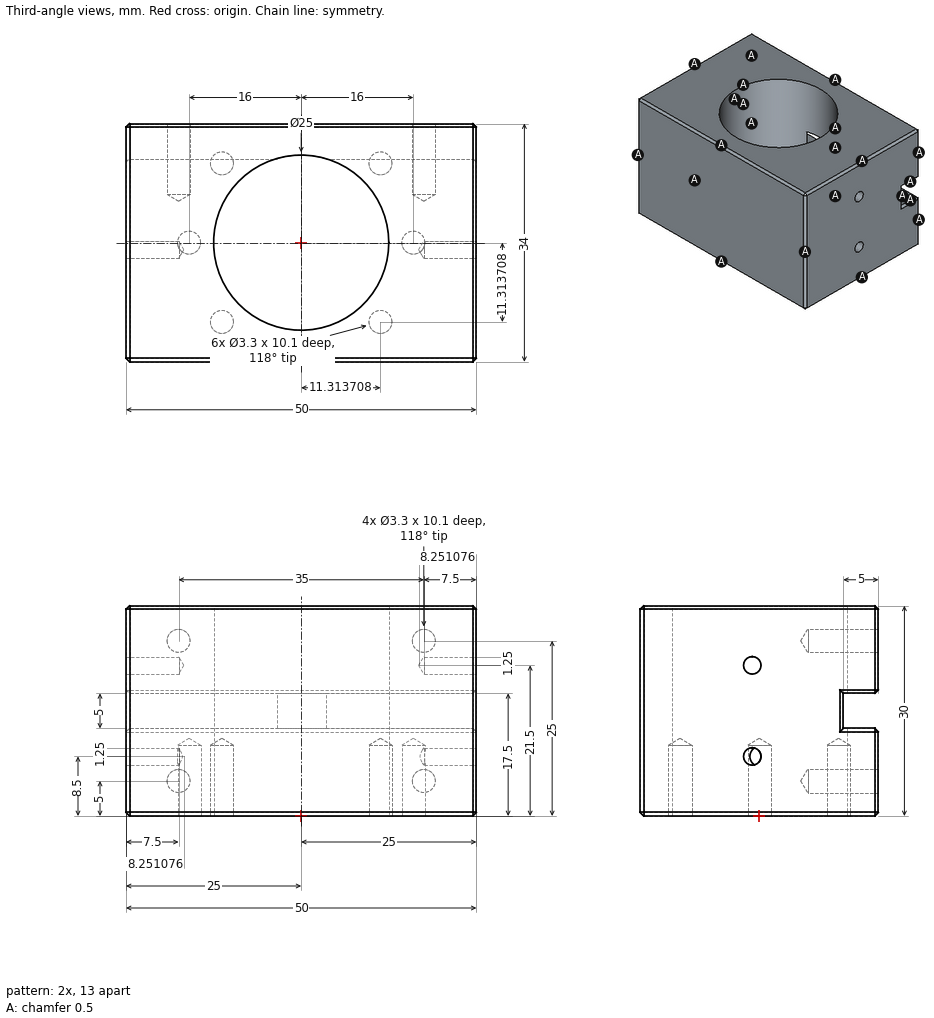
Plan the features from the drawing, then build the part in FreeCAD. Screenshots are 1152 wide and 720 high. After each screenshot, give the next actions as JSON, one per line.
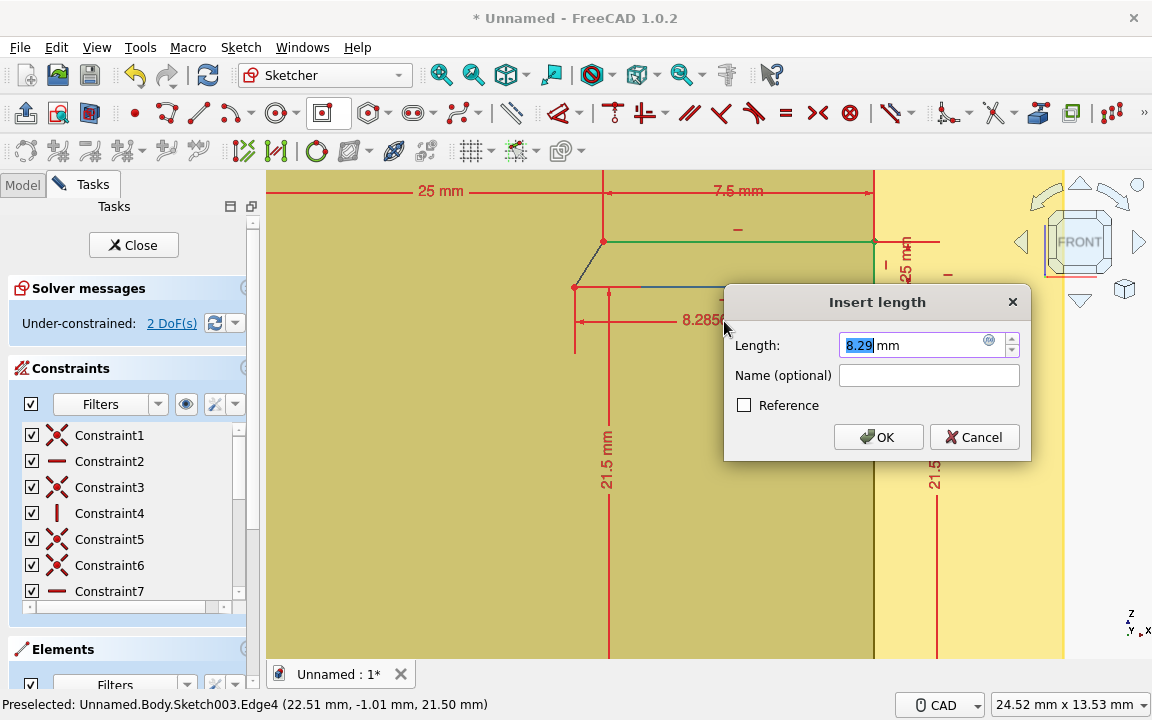
{"action": "type", "text": "8.251076"}
{"action": "key", "text": "Return"}
{"action": "key", "text": "Escape"}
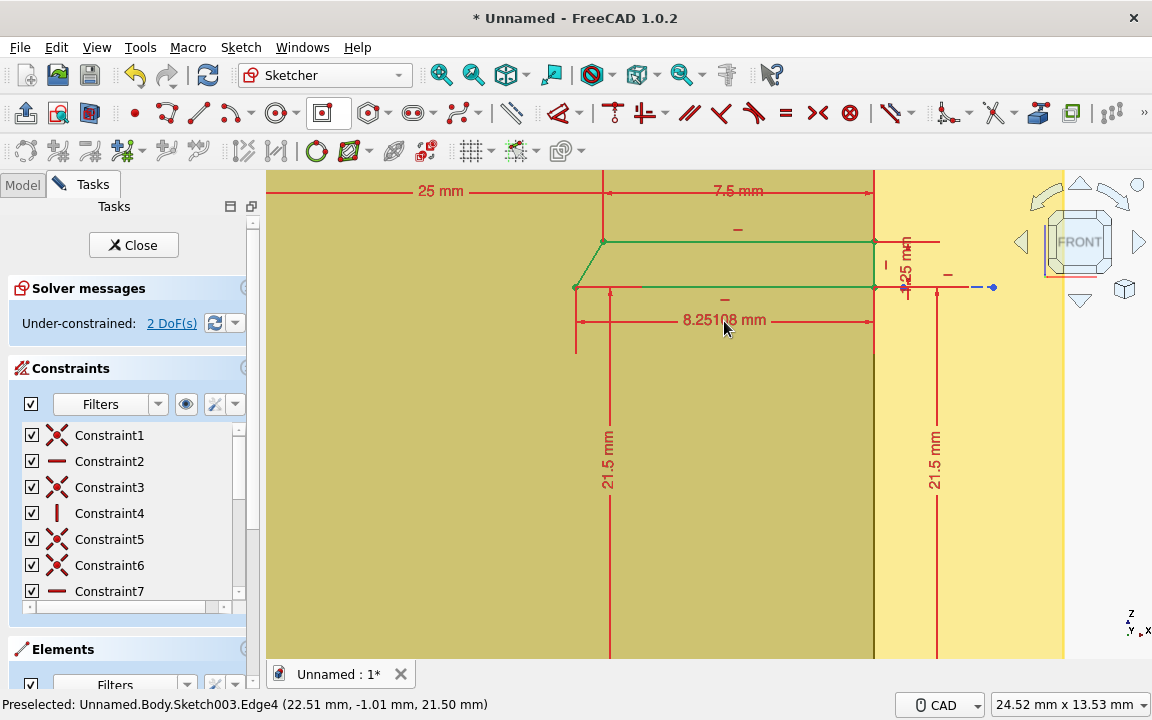
{"action": "left_click", "coordinate": [134, 245]}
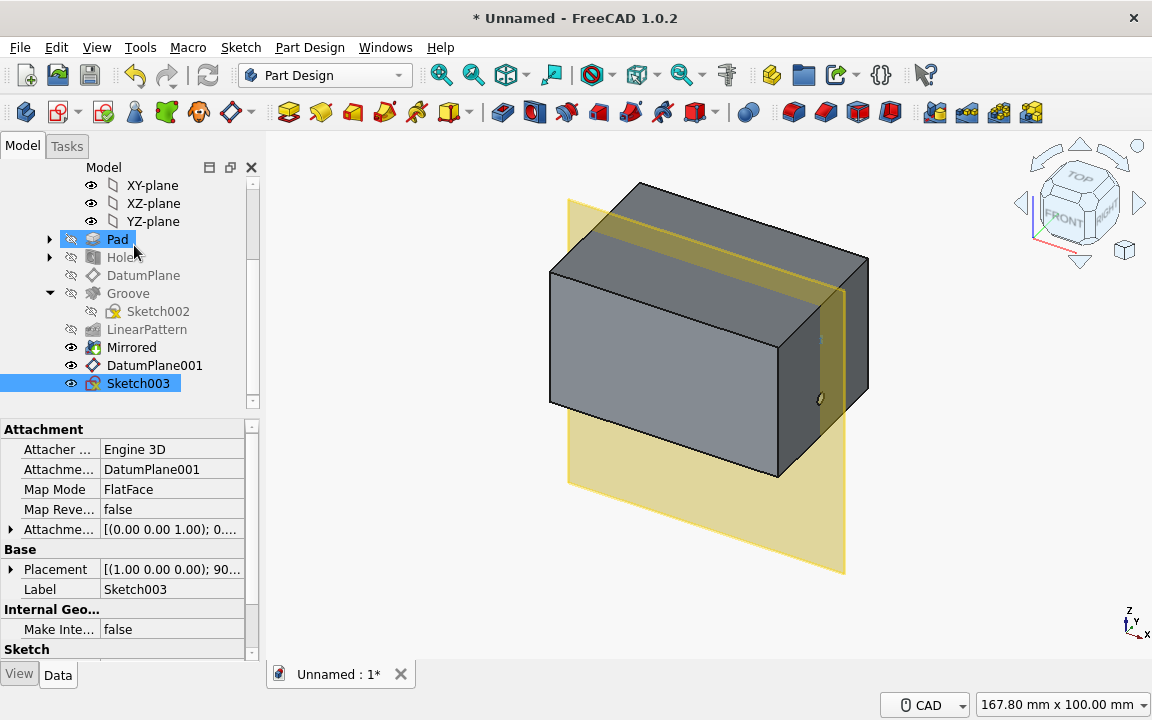
{"action": "left_click", "coordinate": [568, 112]}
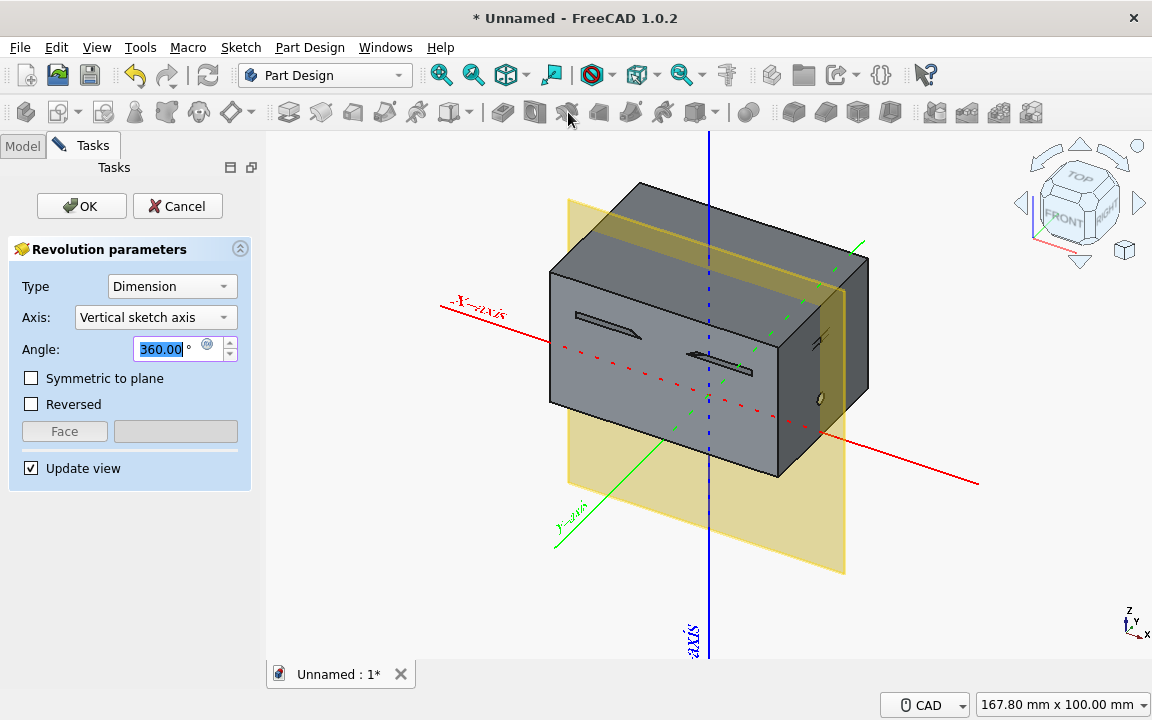
{"action": "left_click", "coordinate": [156, 318]}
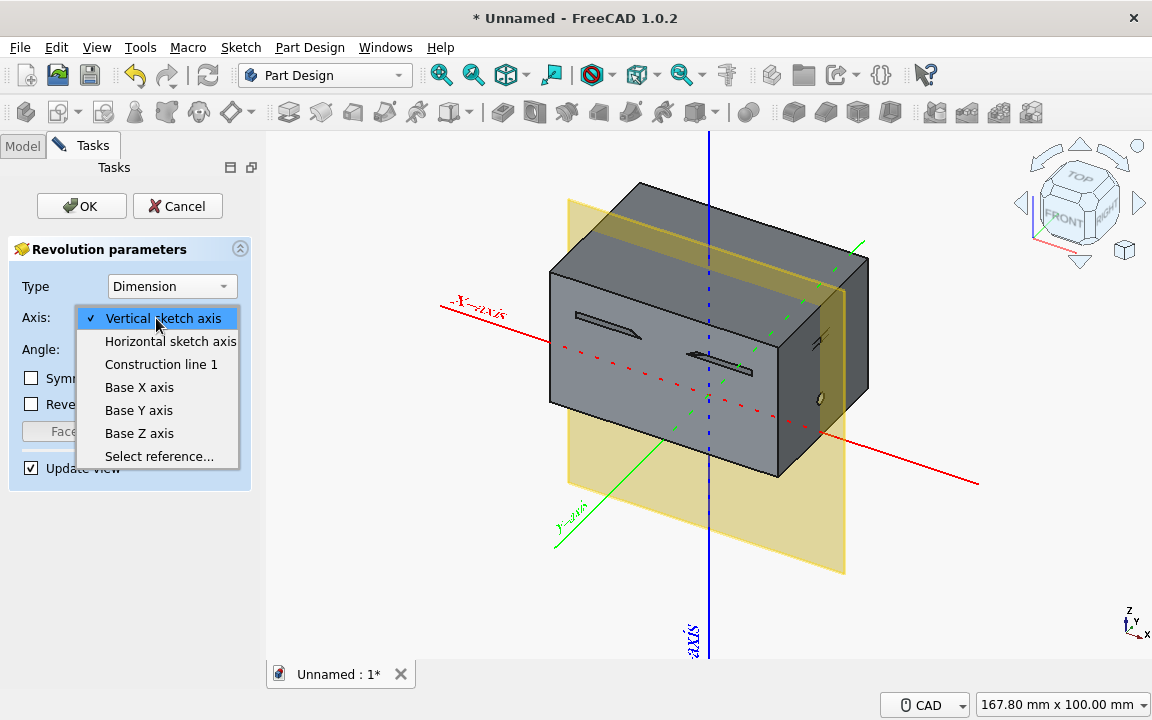
{"action": "left_click", "coordinate": [156, 364]}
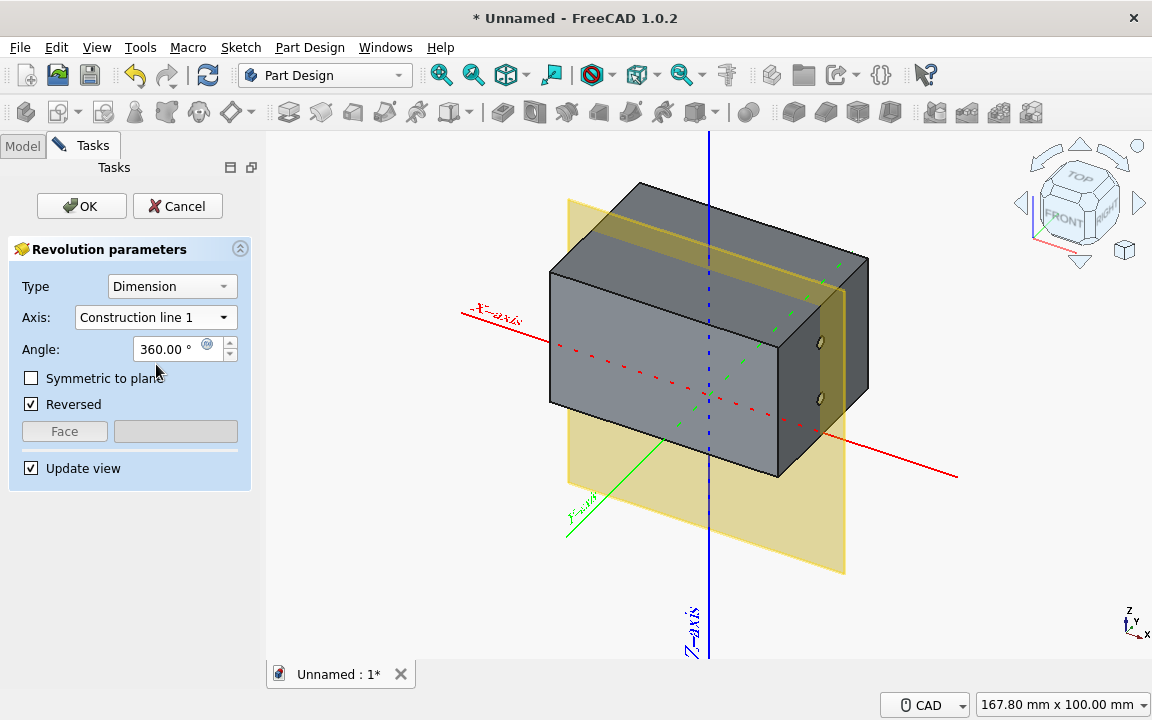
{"action": "left_click", "coordinate": [82, 206]}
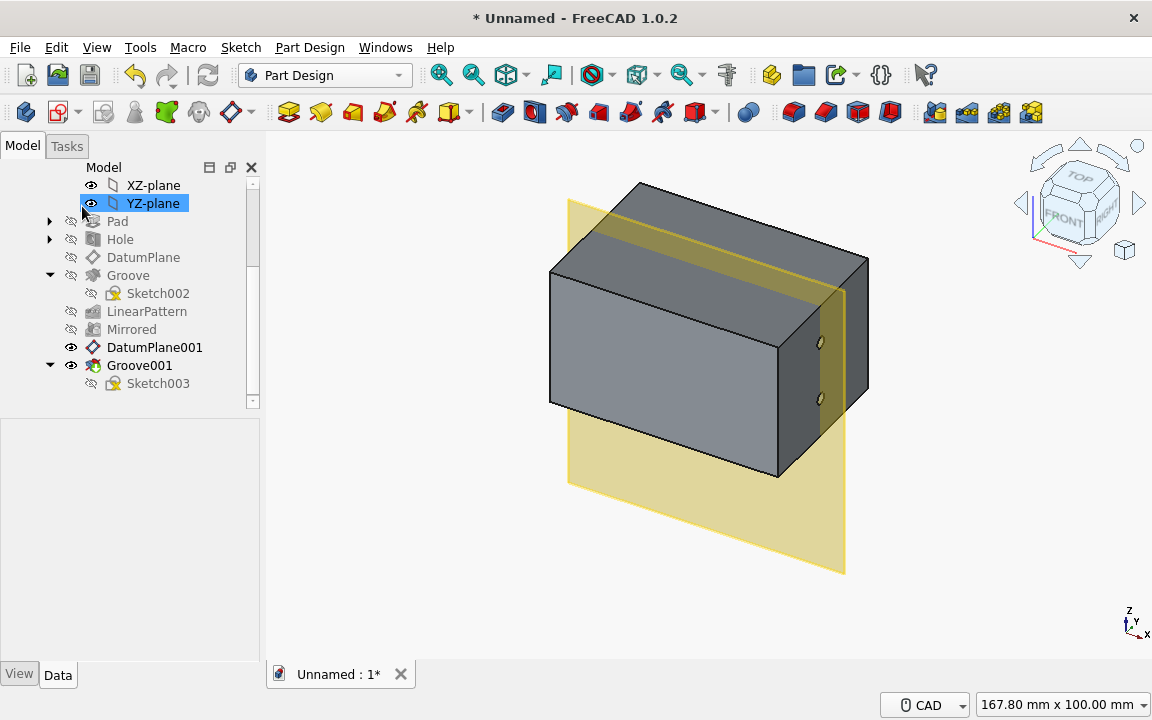
{"action": "left_click", "coordinate": [116, 347]}
{"action": "key", "text": "space"}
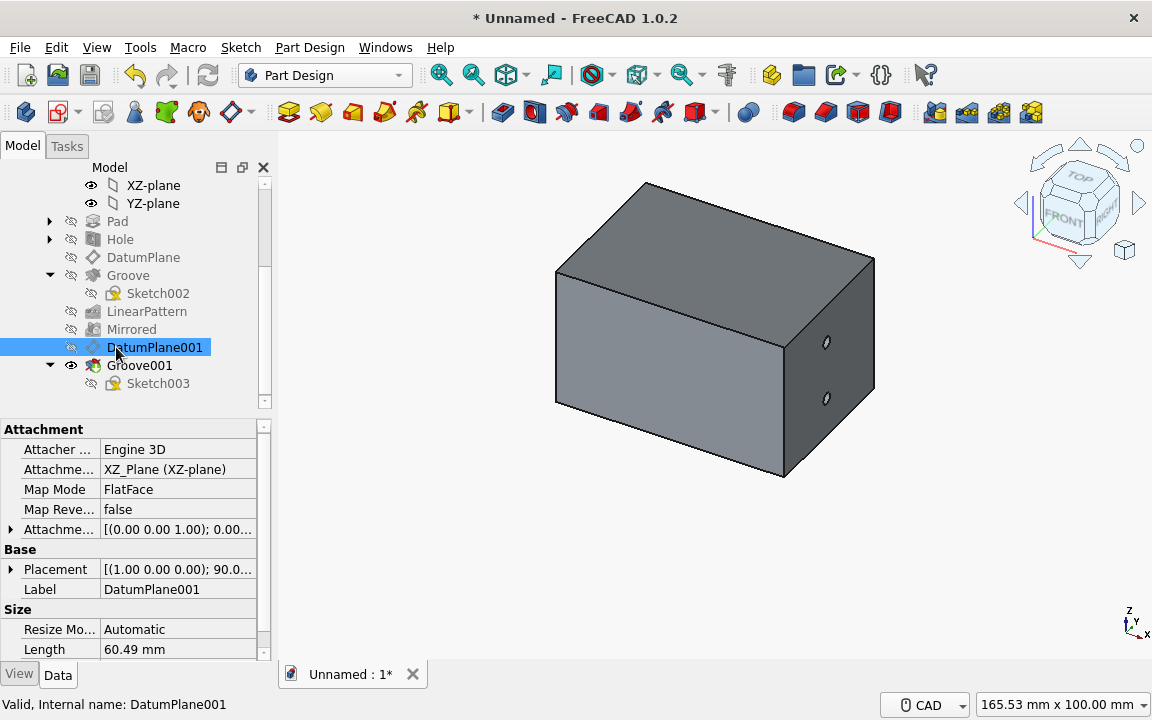
{"action": "left_click", "coordinate": [748, 275]}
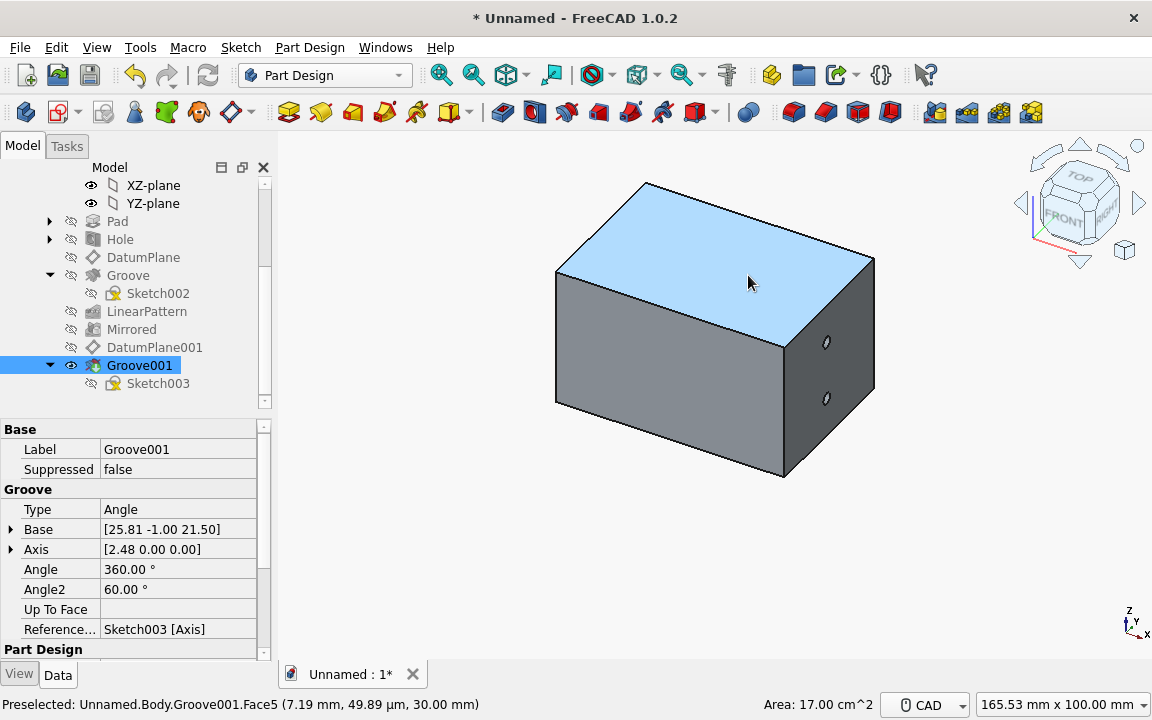
{"action": "left_click", "coordinate": [58, 112]}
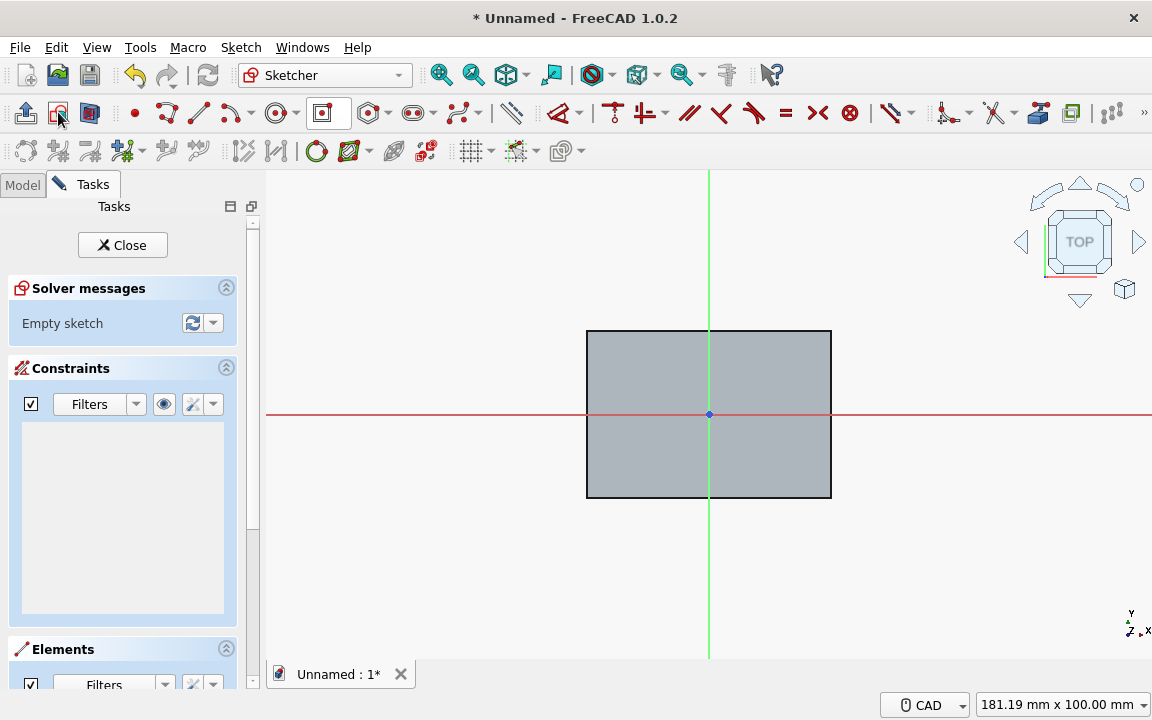
{"action": "scroll", "coordinate": [749, 415], "scroll_direction": "up", "scroll_amount": 5}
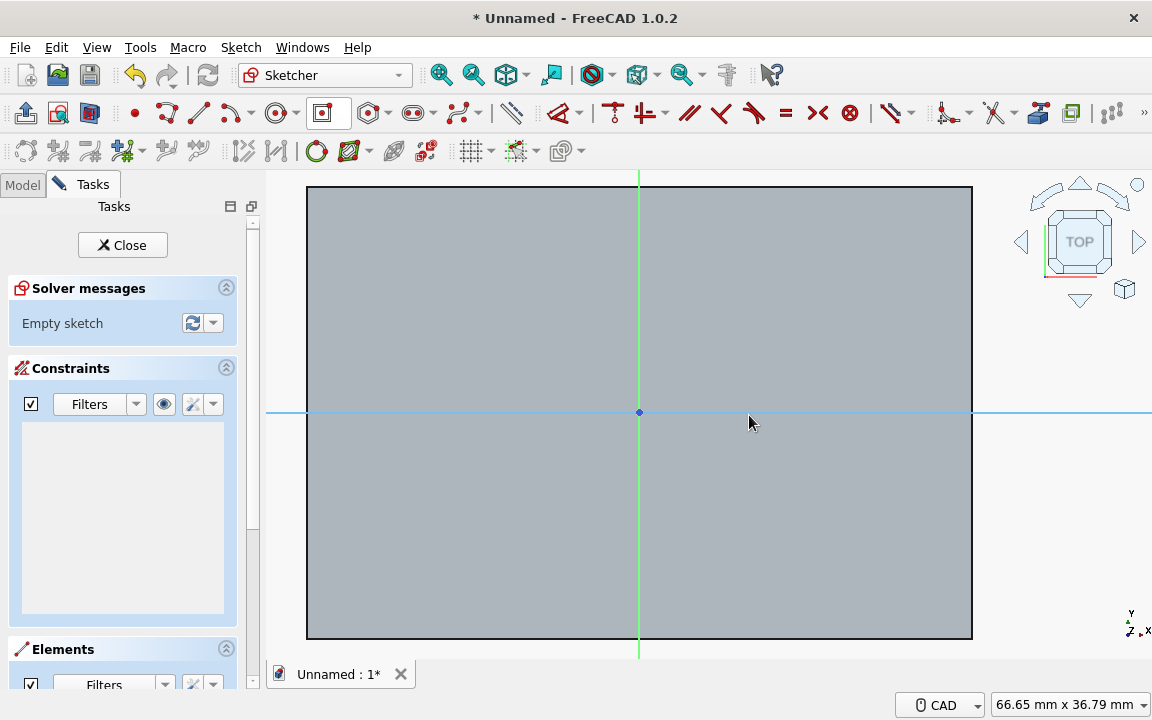
{"action": "left_click", "coordinate": [276, 114]}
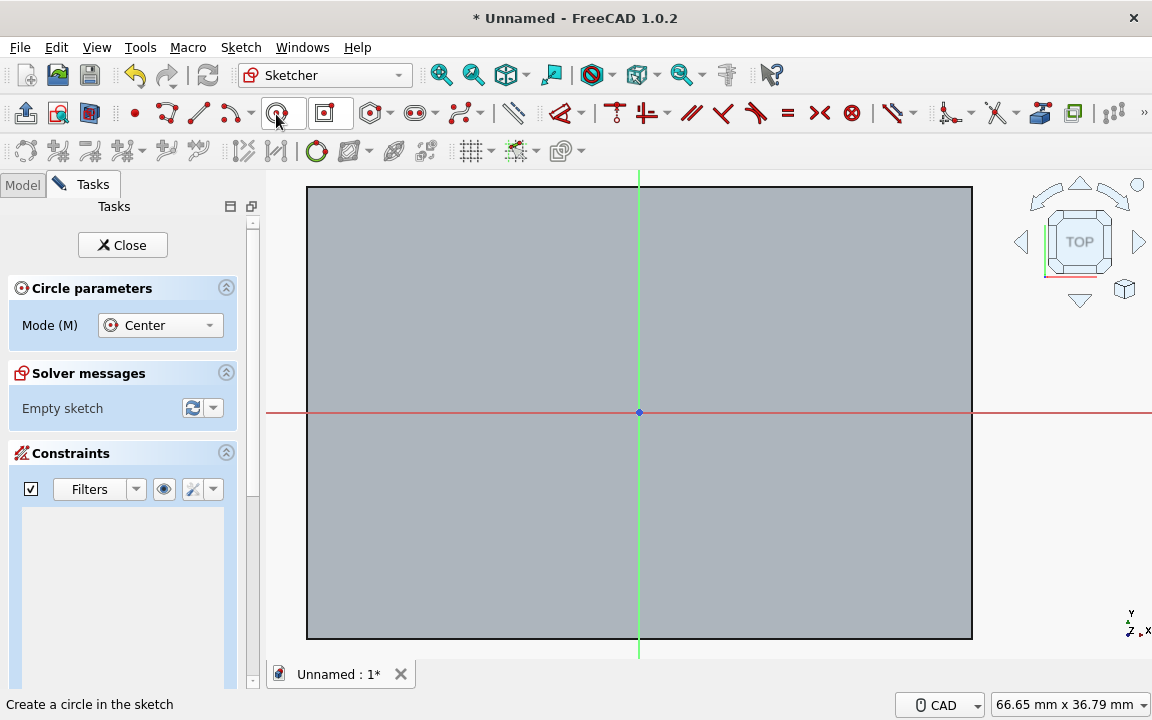
{"action": "left_click", "coordinate": [639, 413]}
{"action": "mouse_move", "coordinate": [757, 295]}